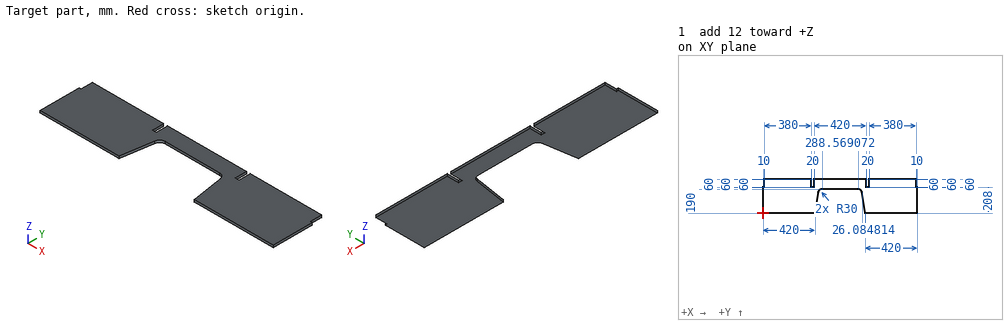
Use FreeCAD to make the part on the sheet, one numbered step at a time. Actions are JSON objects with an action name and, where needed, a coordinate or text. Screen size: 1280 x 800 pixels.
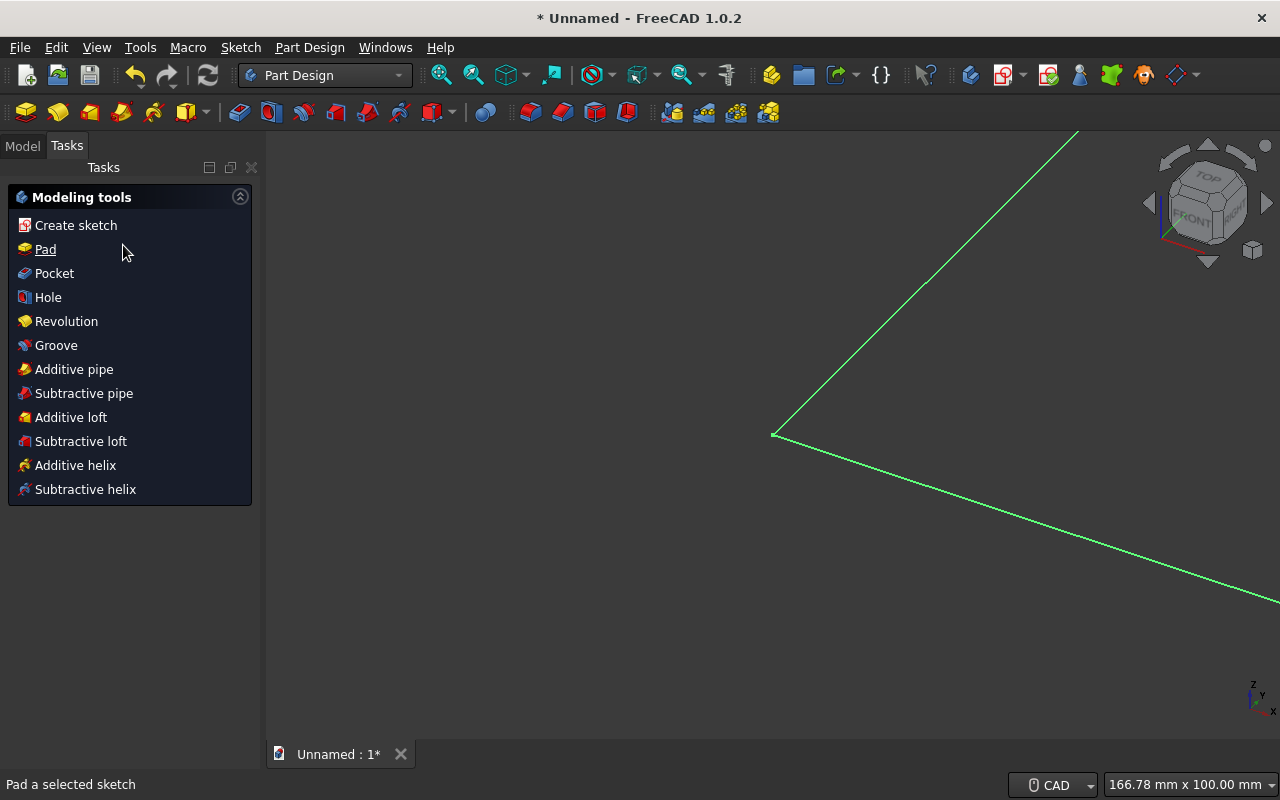
{"action": "left_click", "coordinate": [26, 112]}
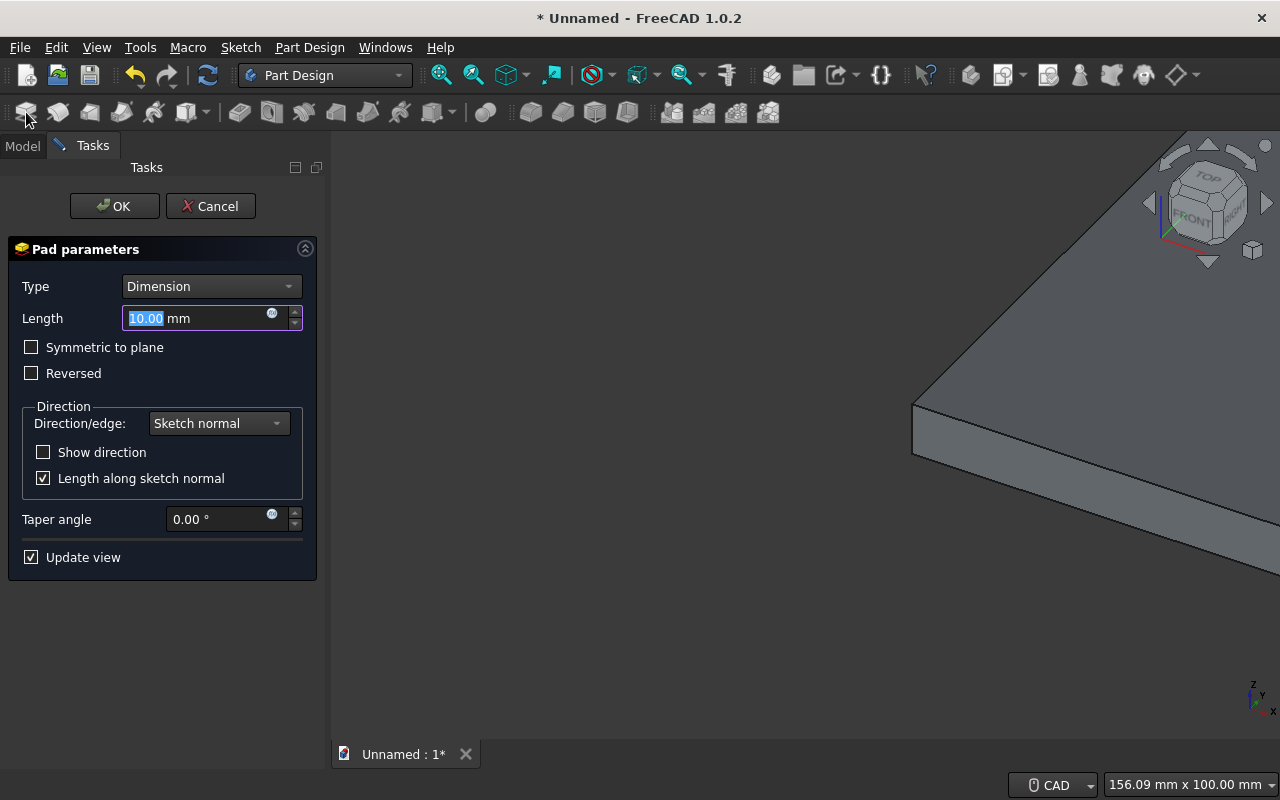
{"action": "type", "text": "12"}
{"action": "key", "text": "Tab"}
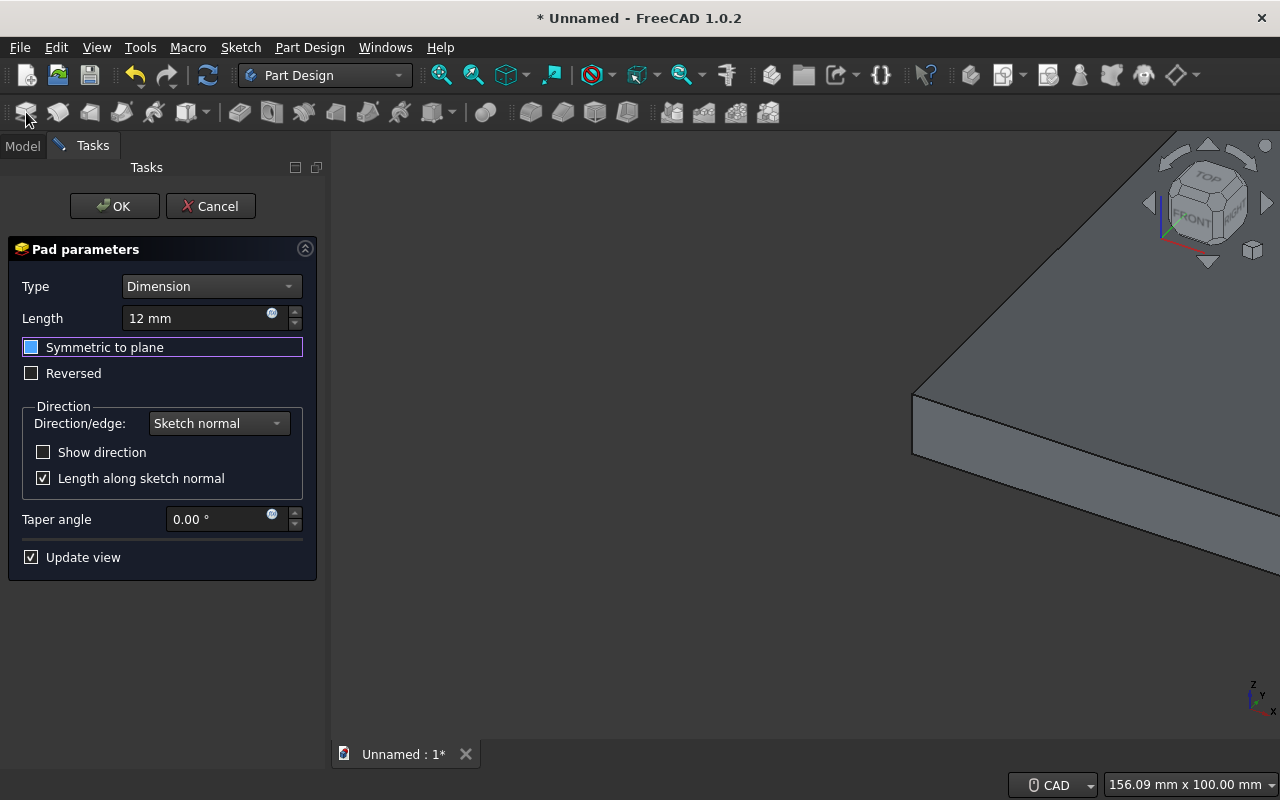
{"action": "left_click", "coordinate": [115, 206]}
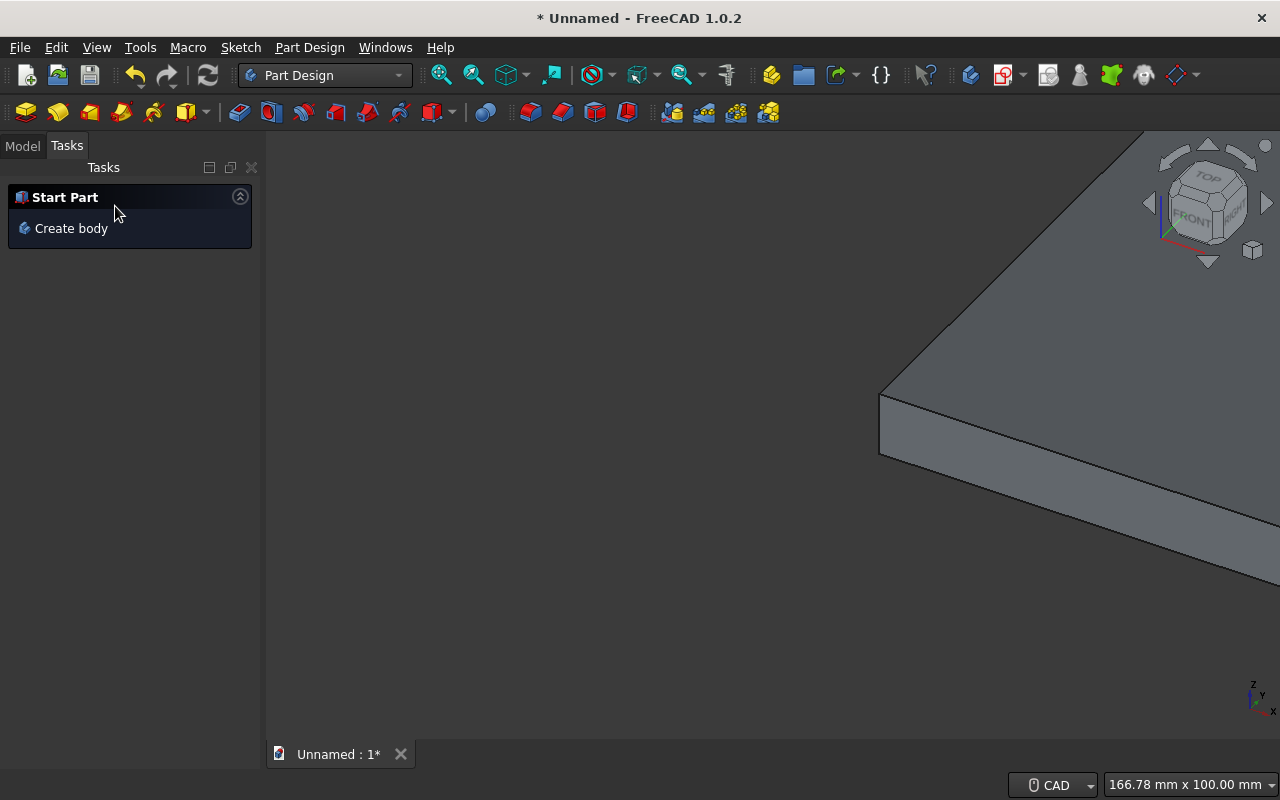
{"action": "key", "text": "0"}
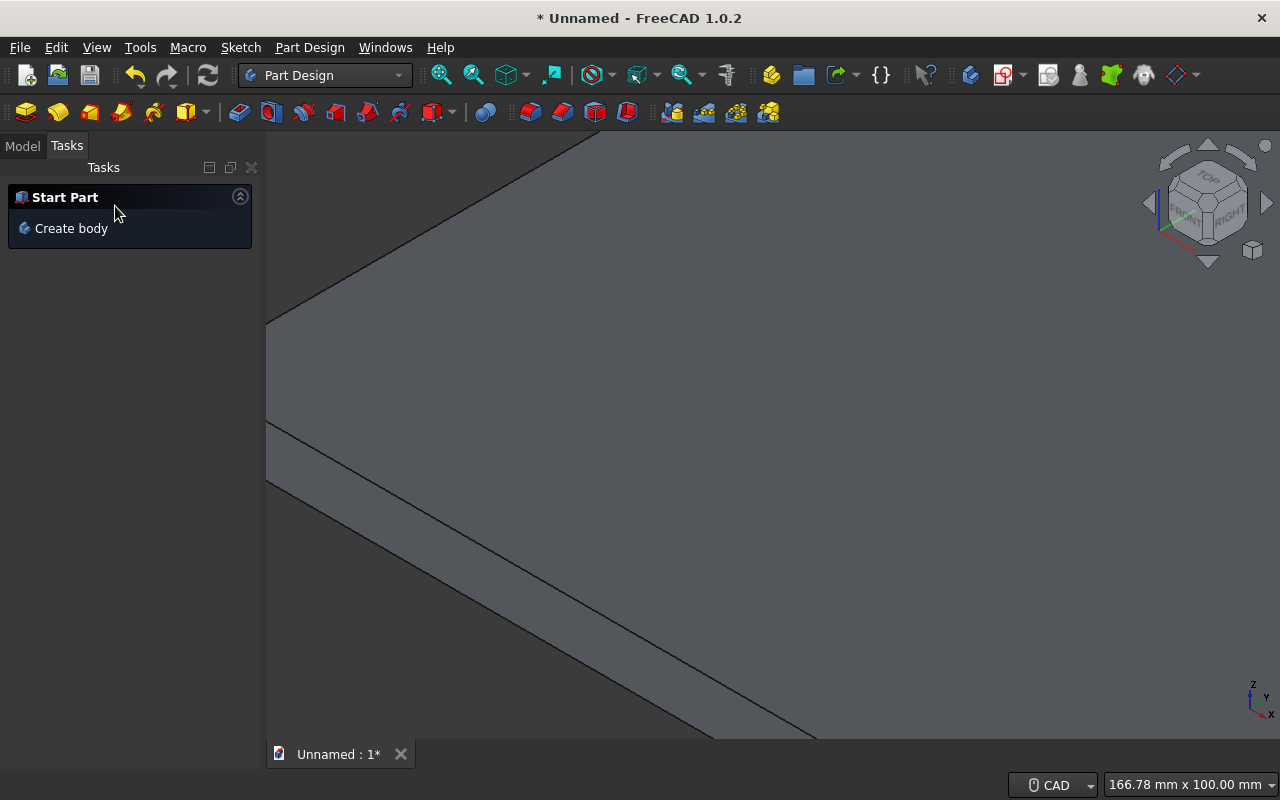
{"action": "left_click", "coordinate": [442, 76]}